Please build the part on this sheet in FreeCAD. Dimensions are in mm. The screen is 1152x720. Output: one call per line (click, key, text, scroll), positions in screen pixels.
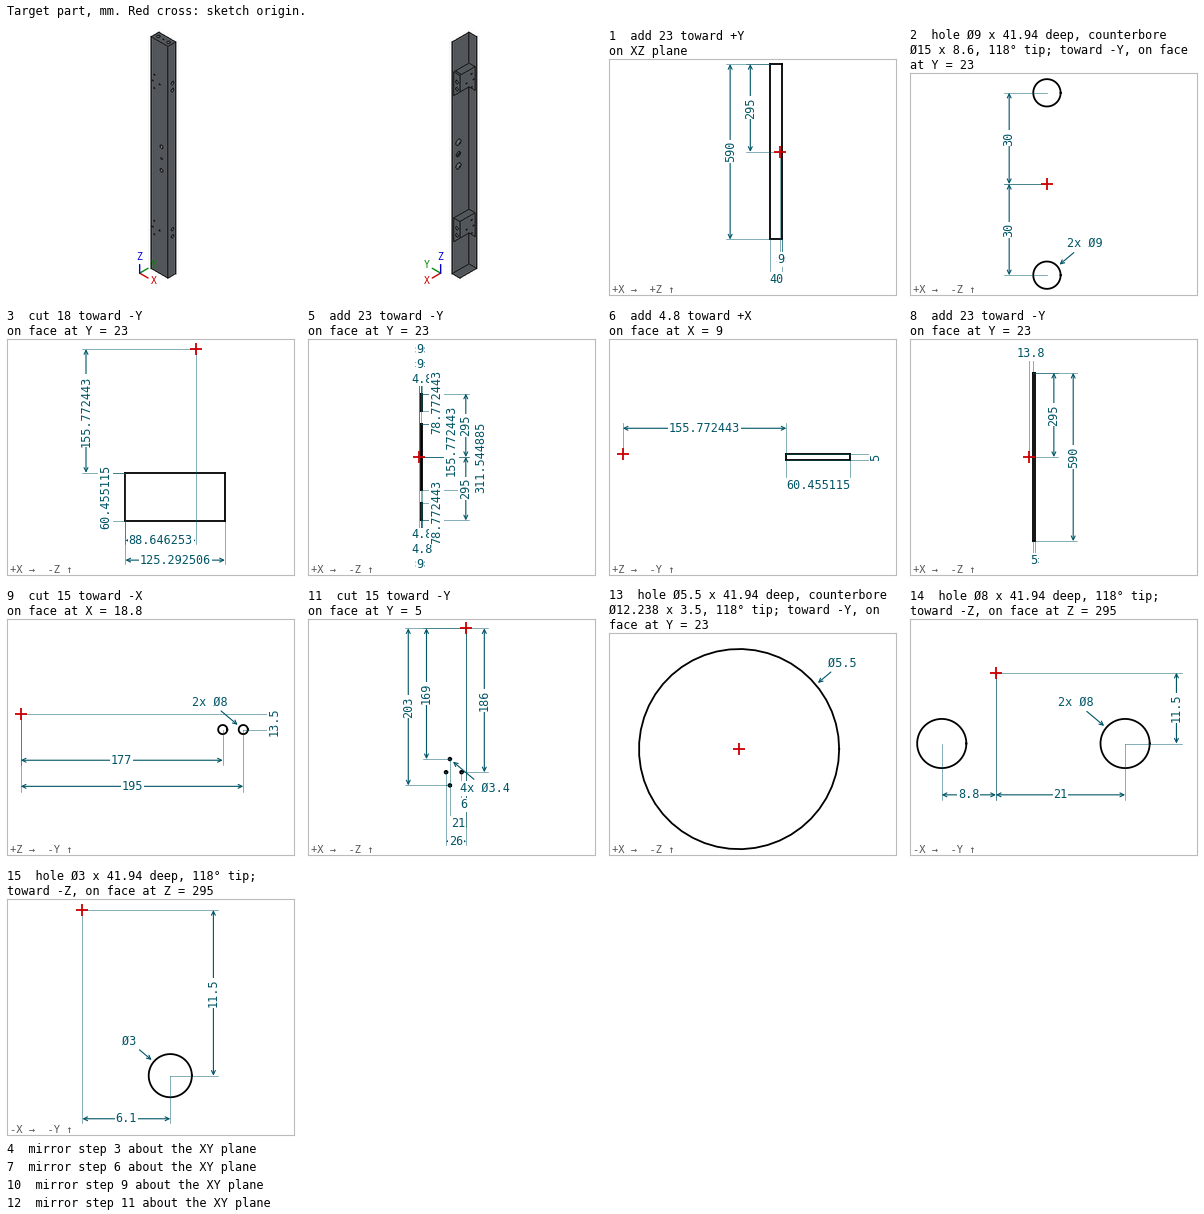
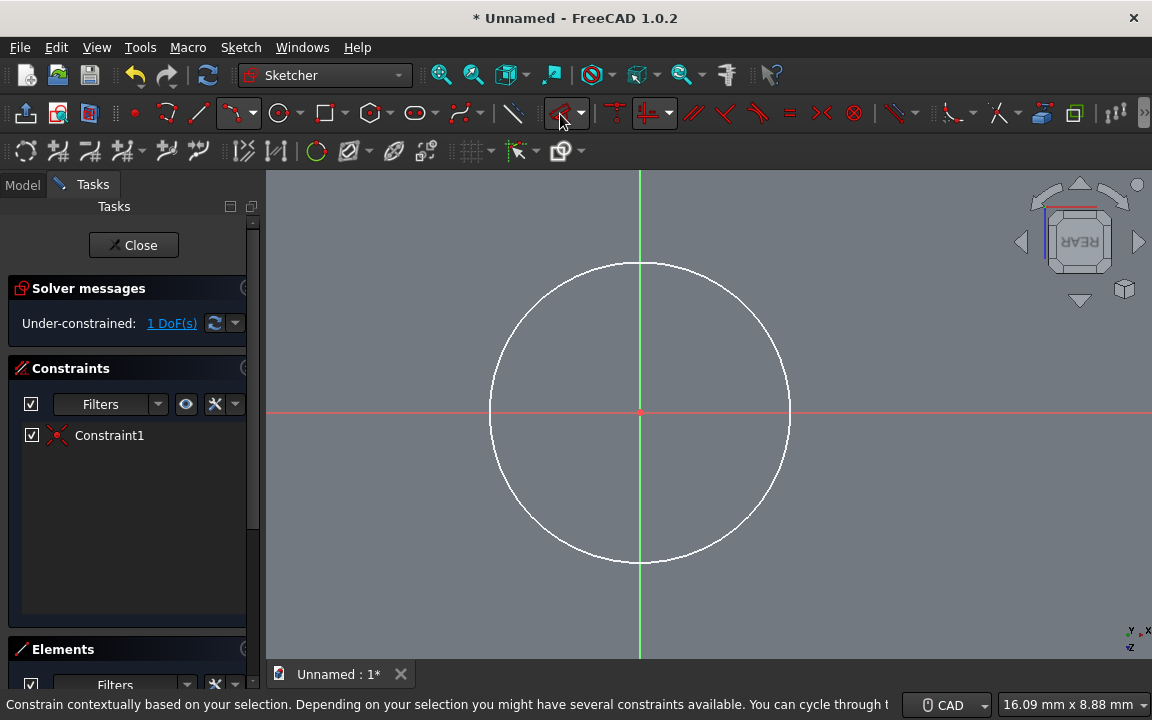
click(746, 306)
click(769, 283)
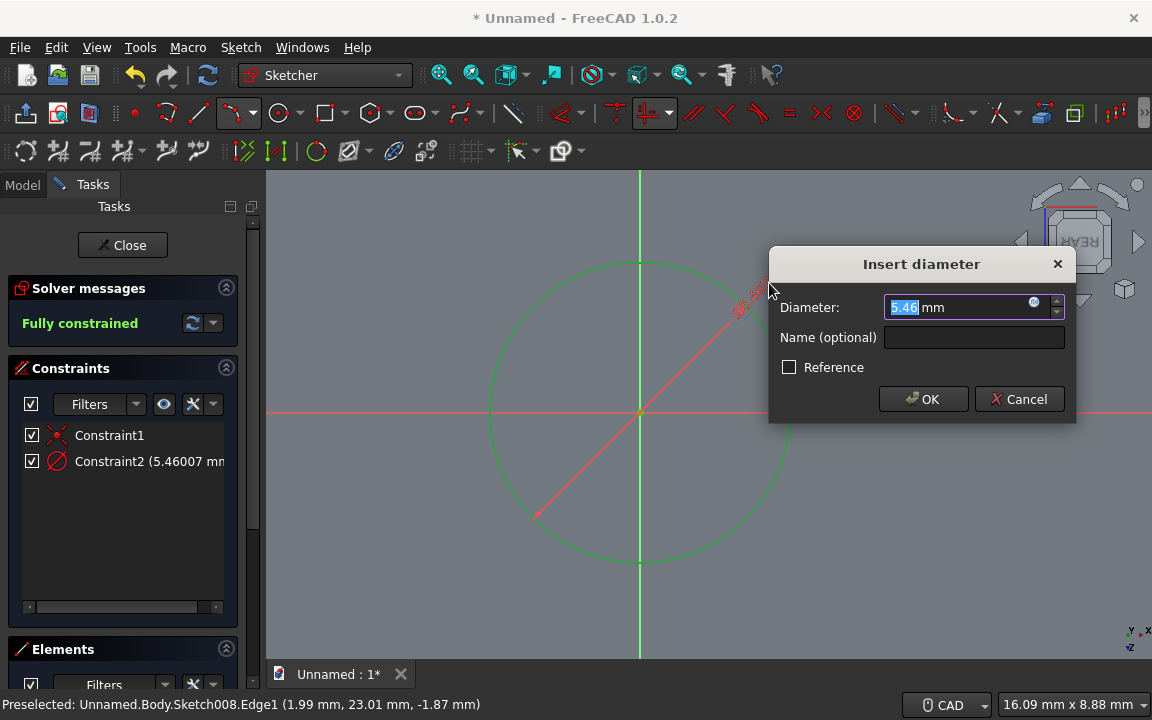
text(5.5)
key(Return)
key(Escape)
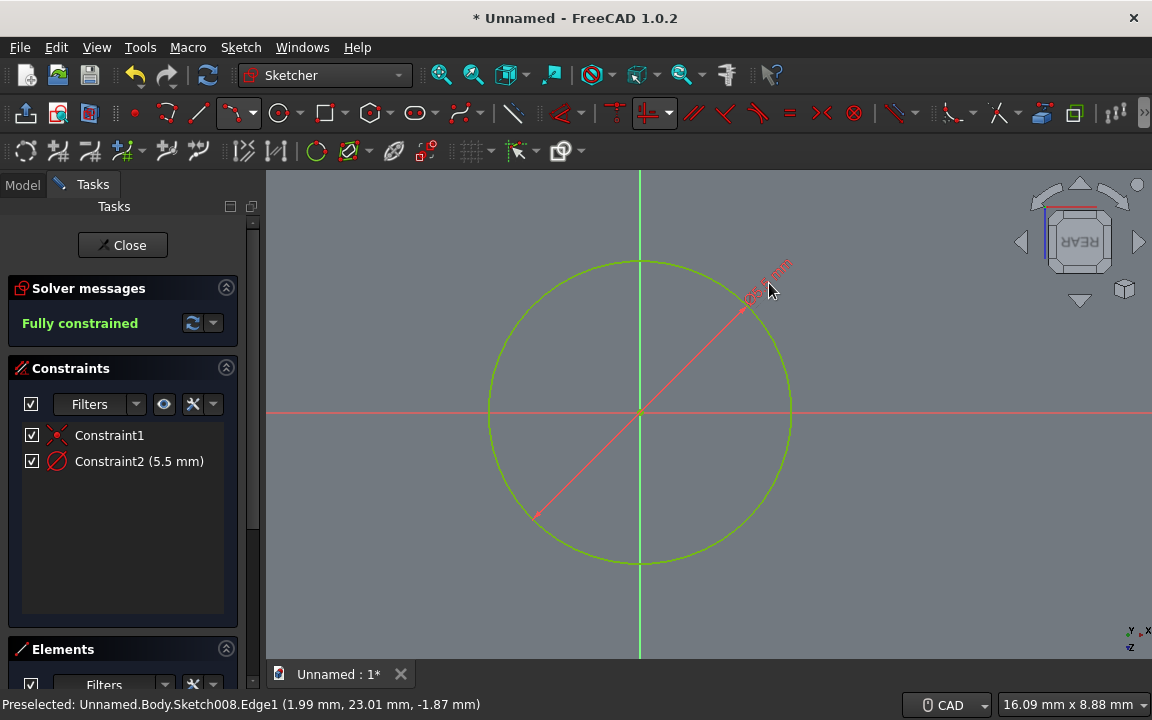
click(123, 245)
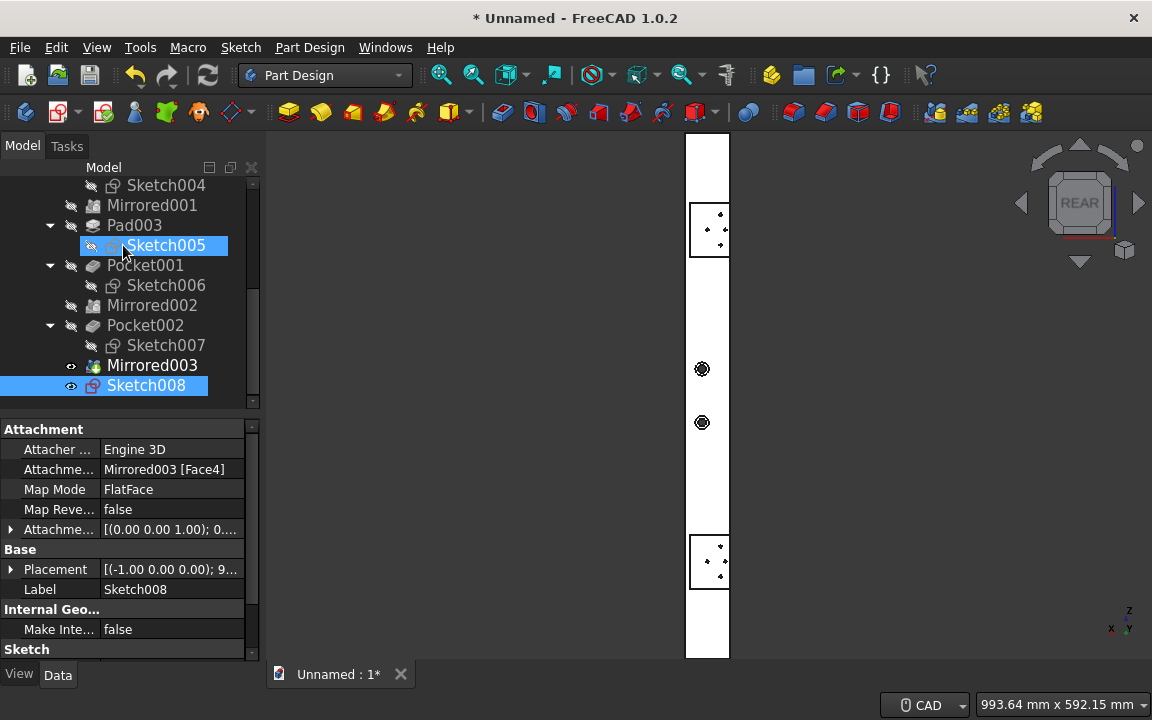
click(536, 112)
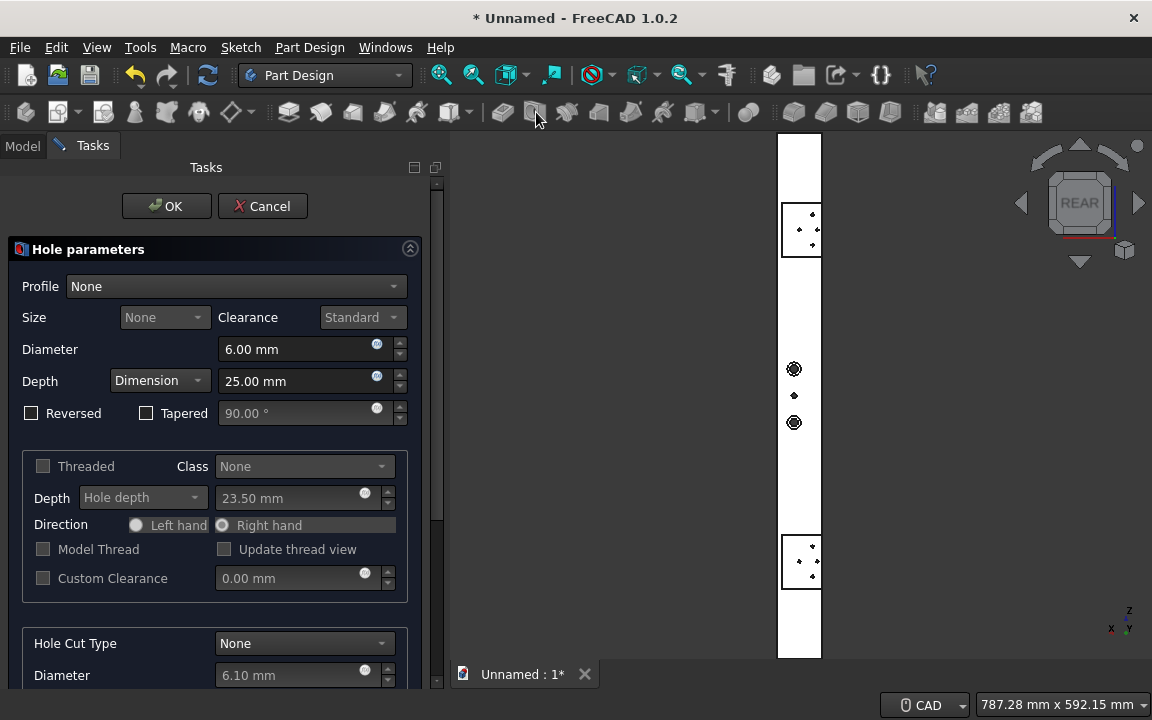
triple_click(305, 349)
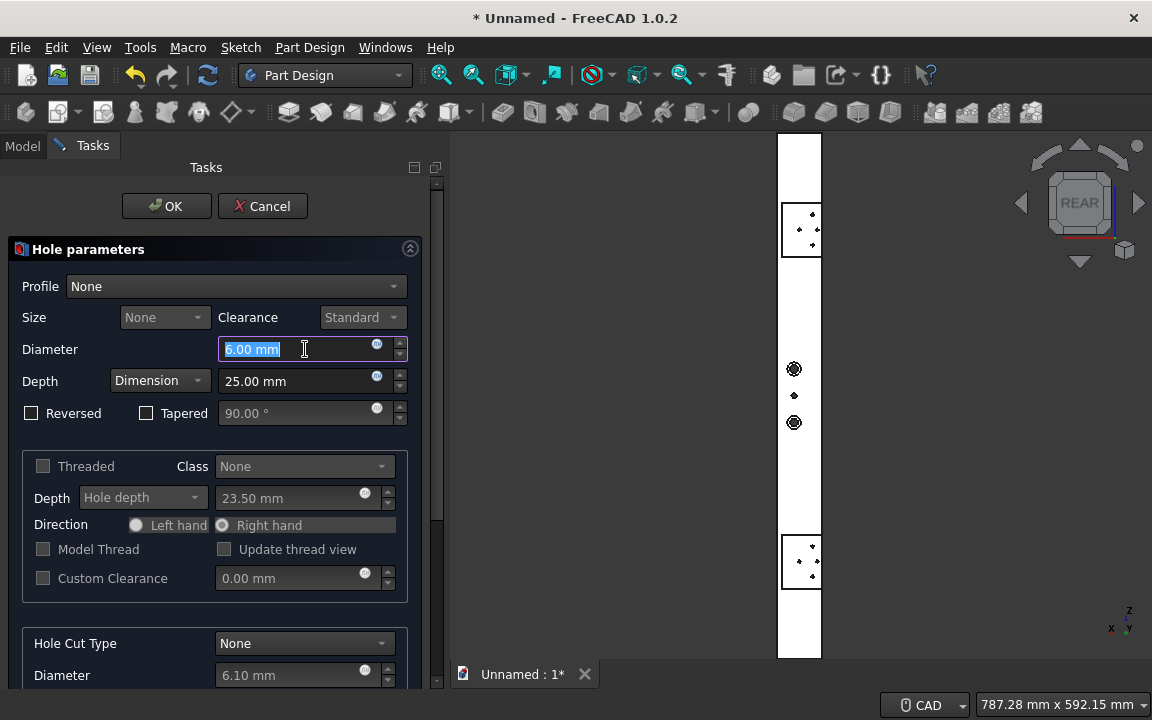
text(5.5)
key(Tab)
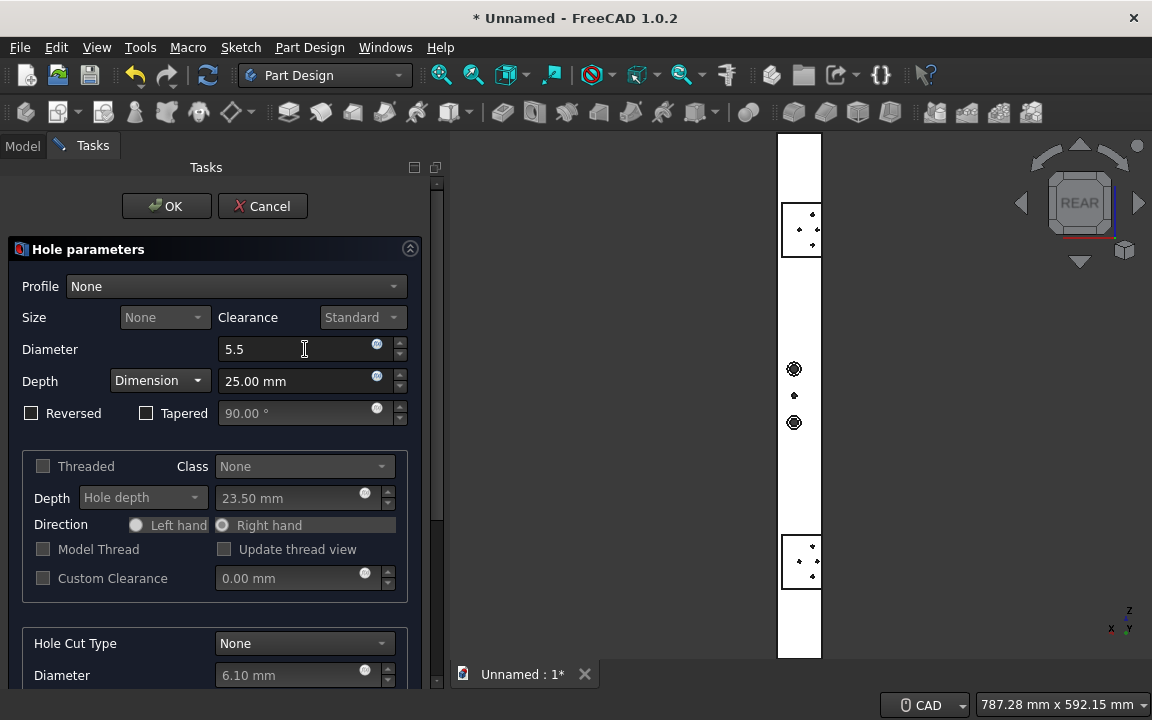
triple_click(305, 381)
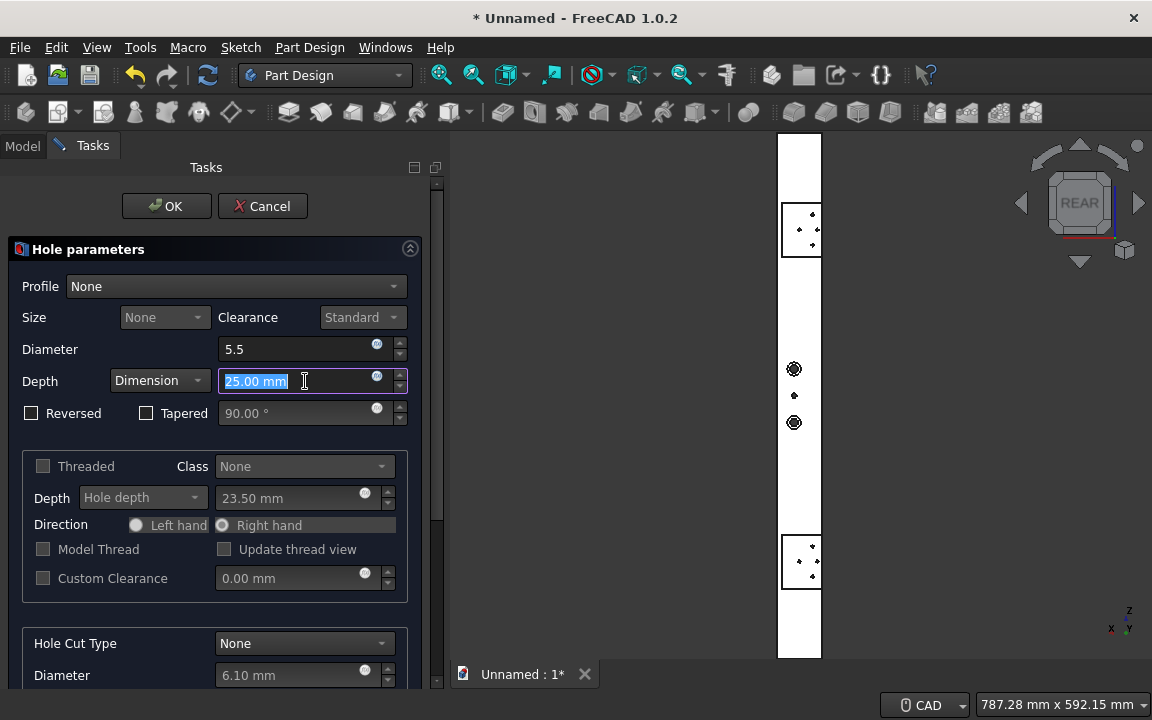
text(41.94)
key(Tab)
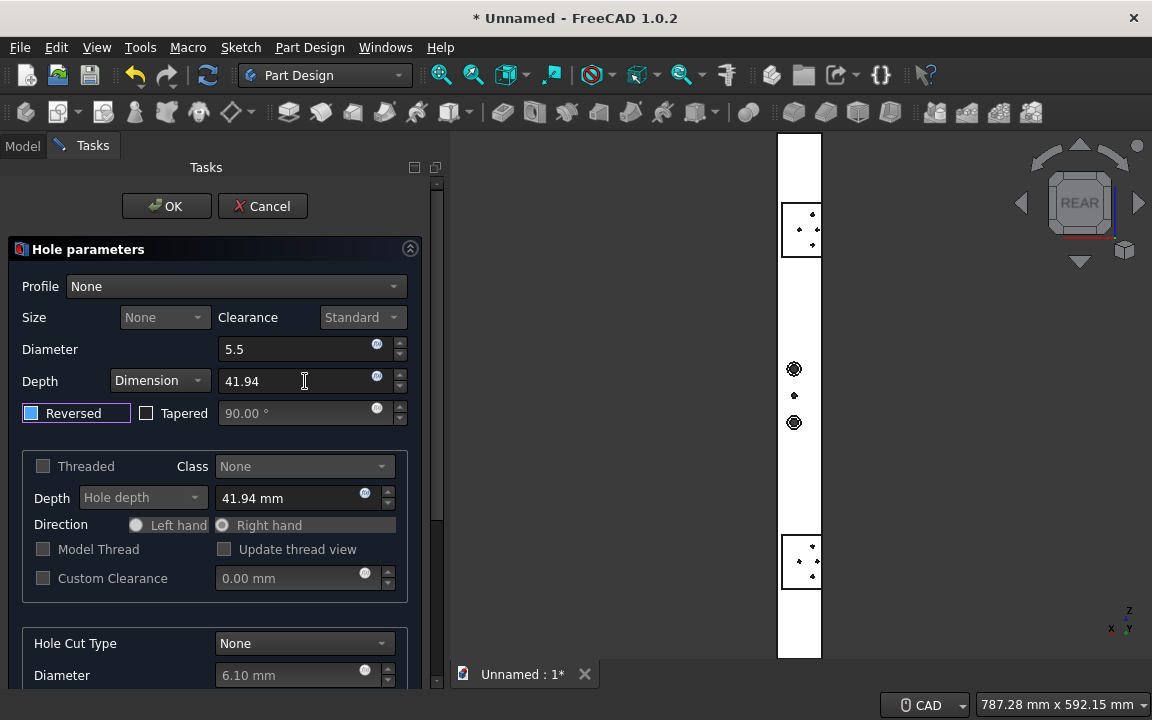
click(306, 644)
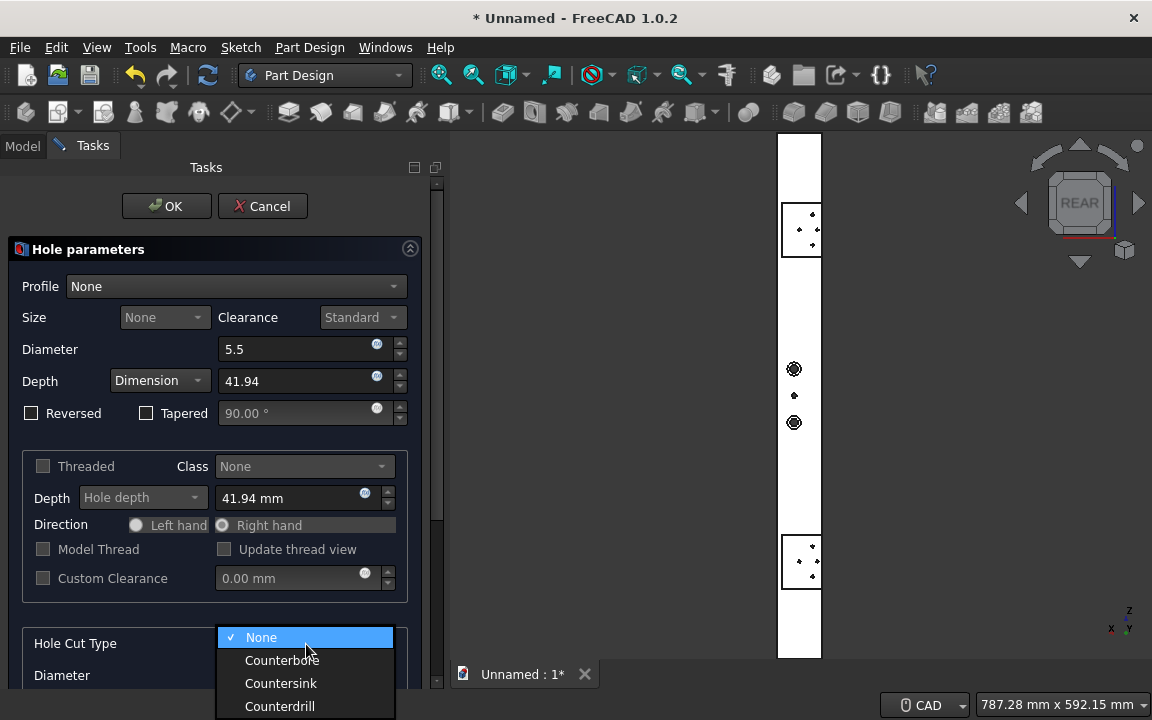
click(304, 660)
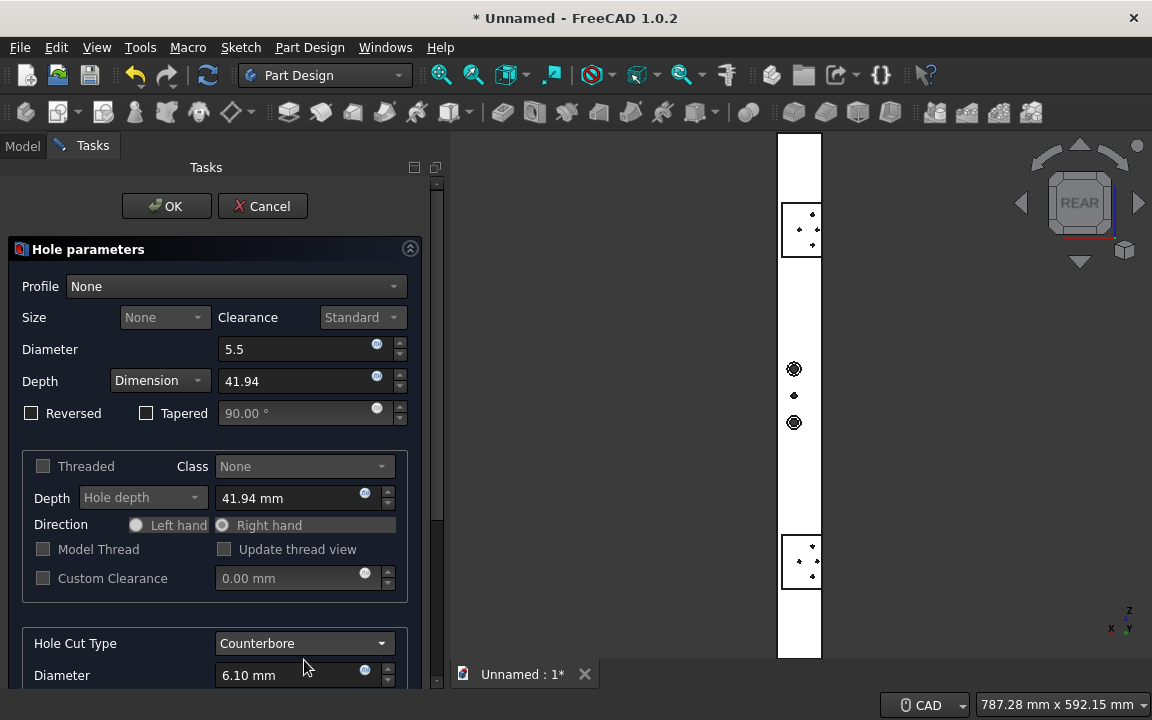
triple_click(298, 675)